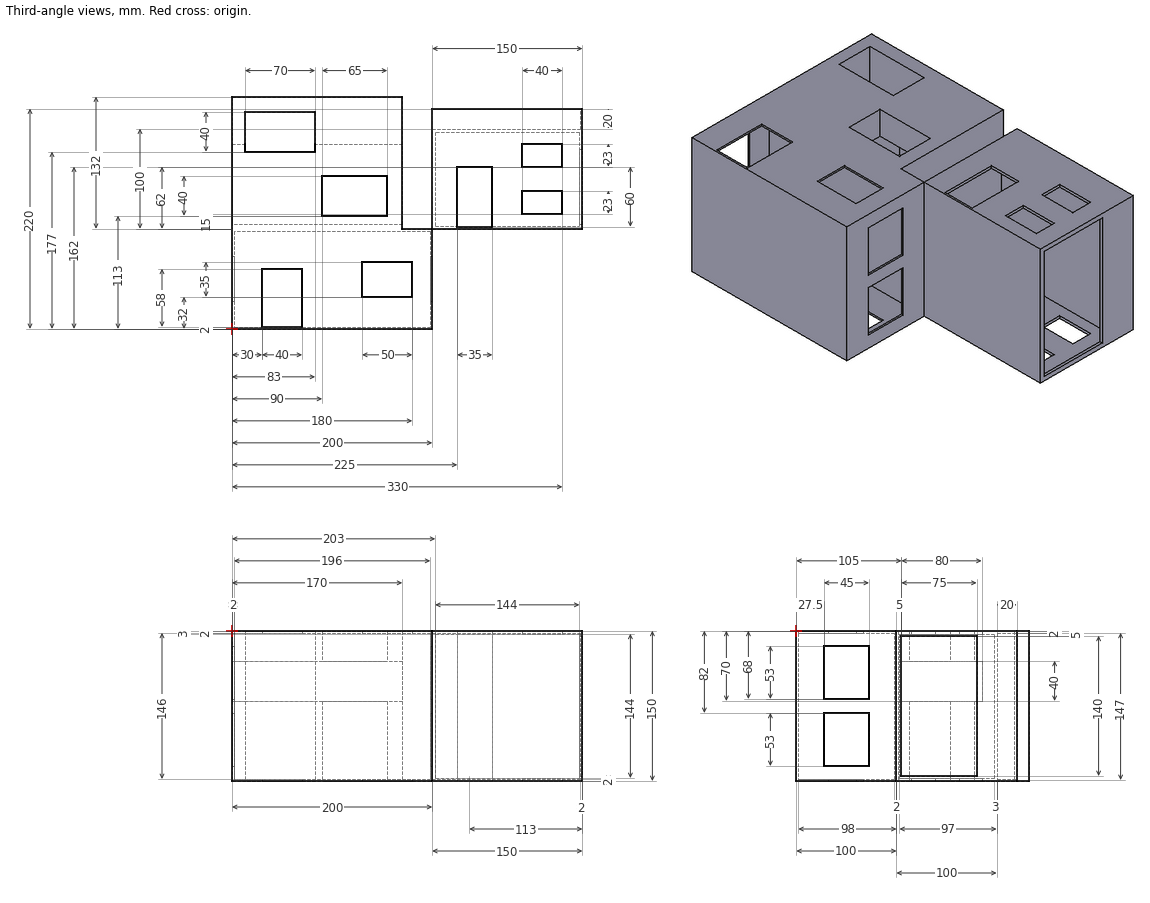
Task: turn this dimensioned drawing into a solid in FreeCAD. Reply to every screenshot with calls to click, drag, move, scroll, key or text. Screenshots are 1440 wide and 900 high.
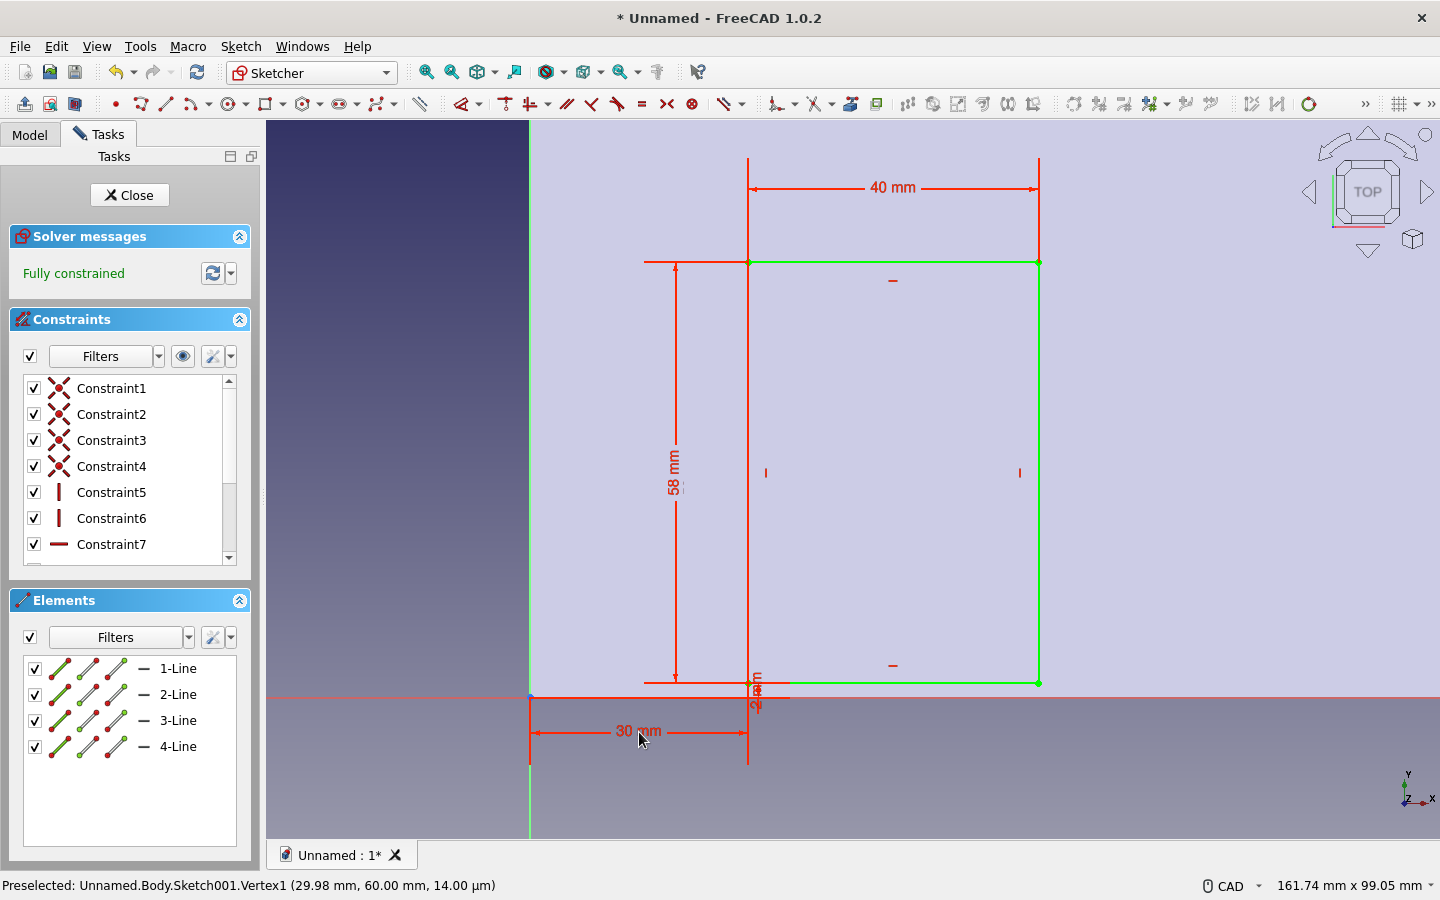
click(130, 195)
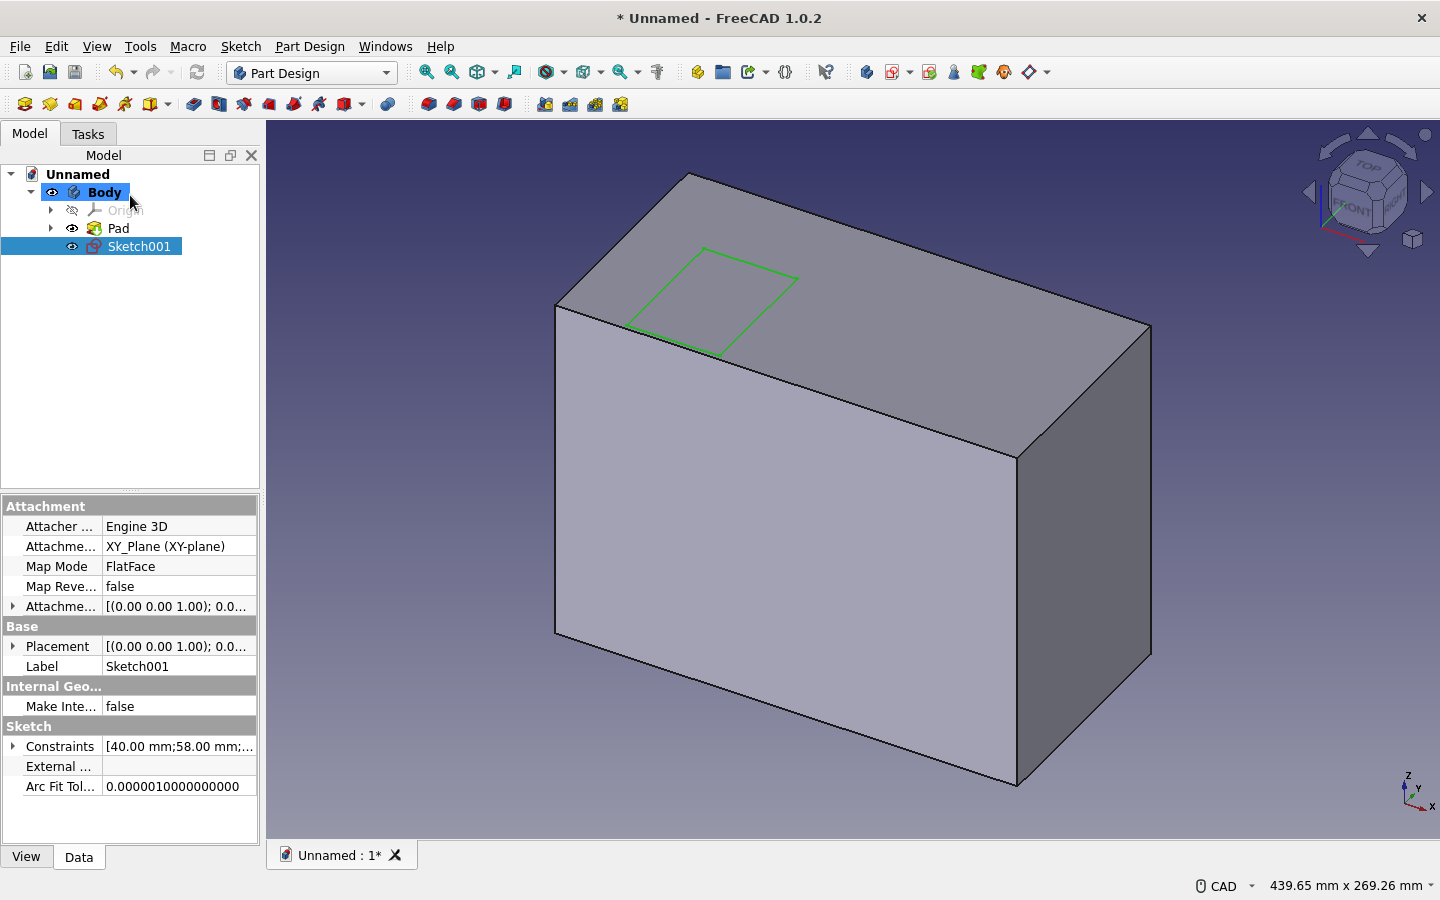
click(194, 104)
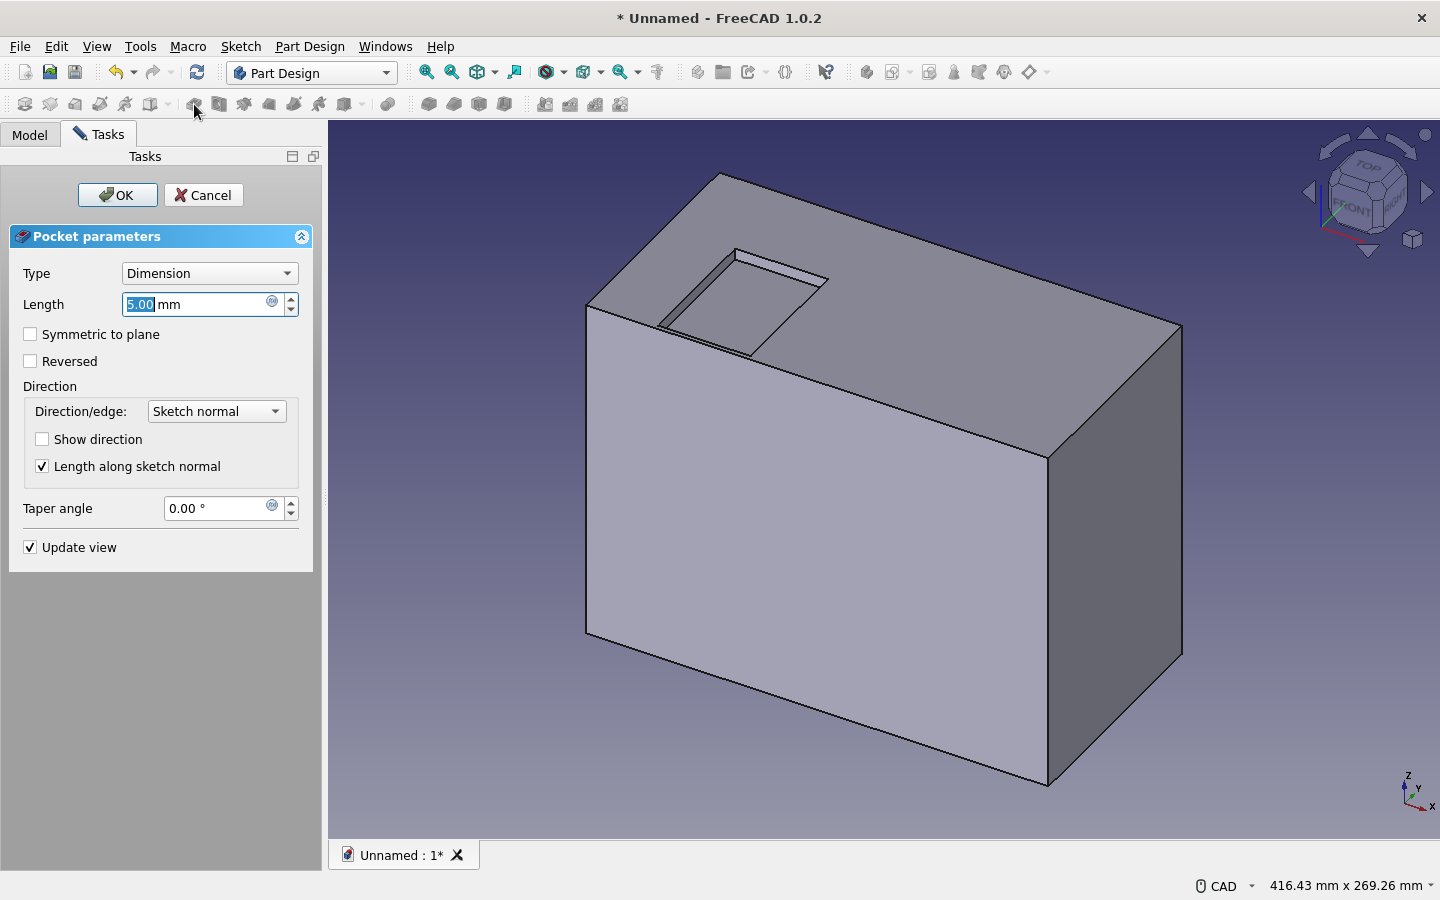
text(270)
key(Tab)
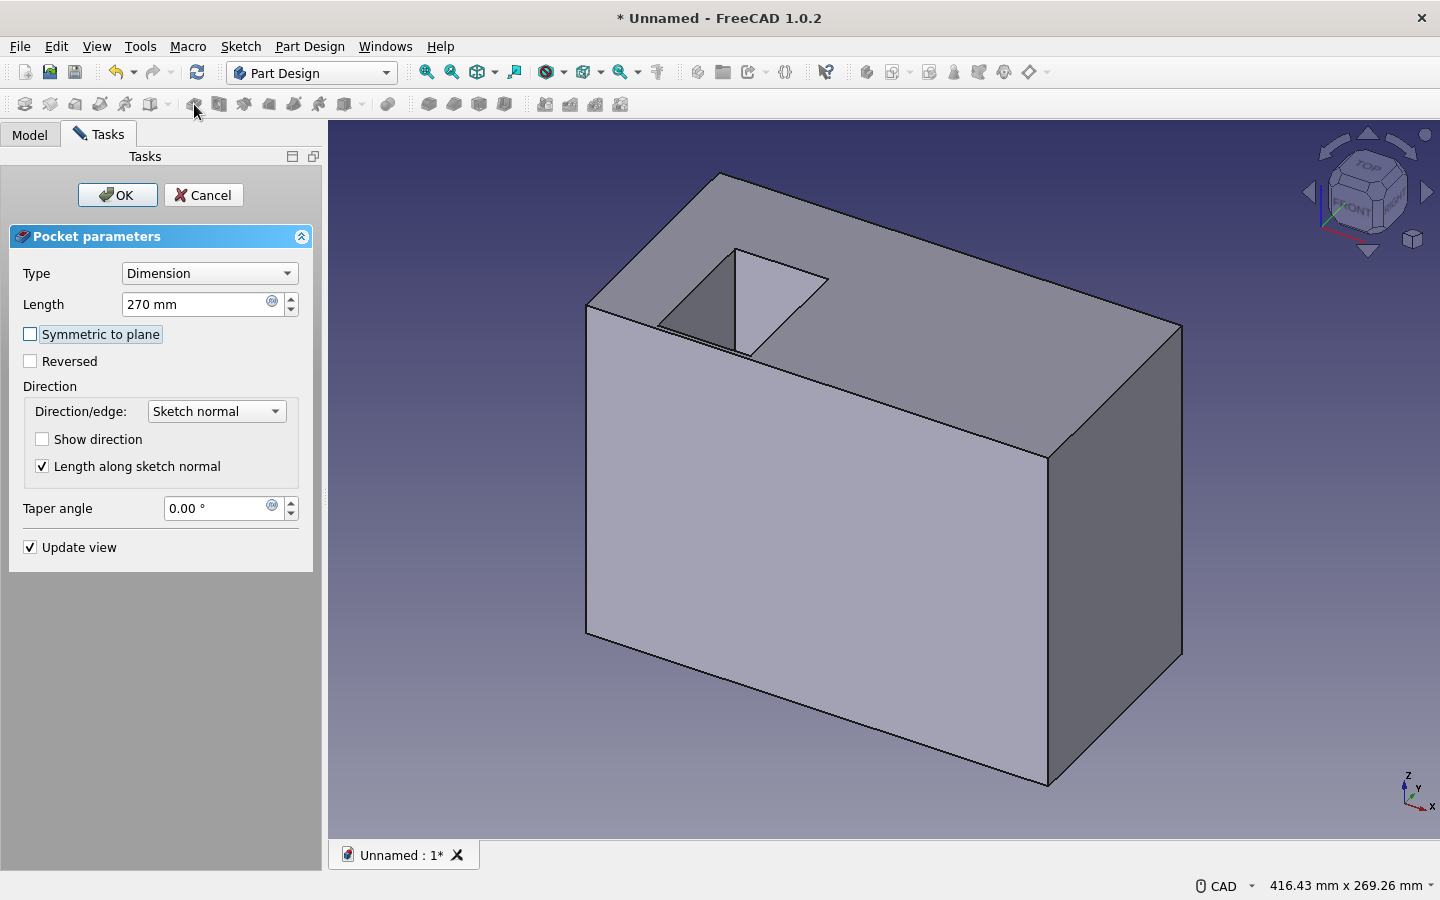
click(118, 195)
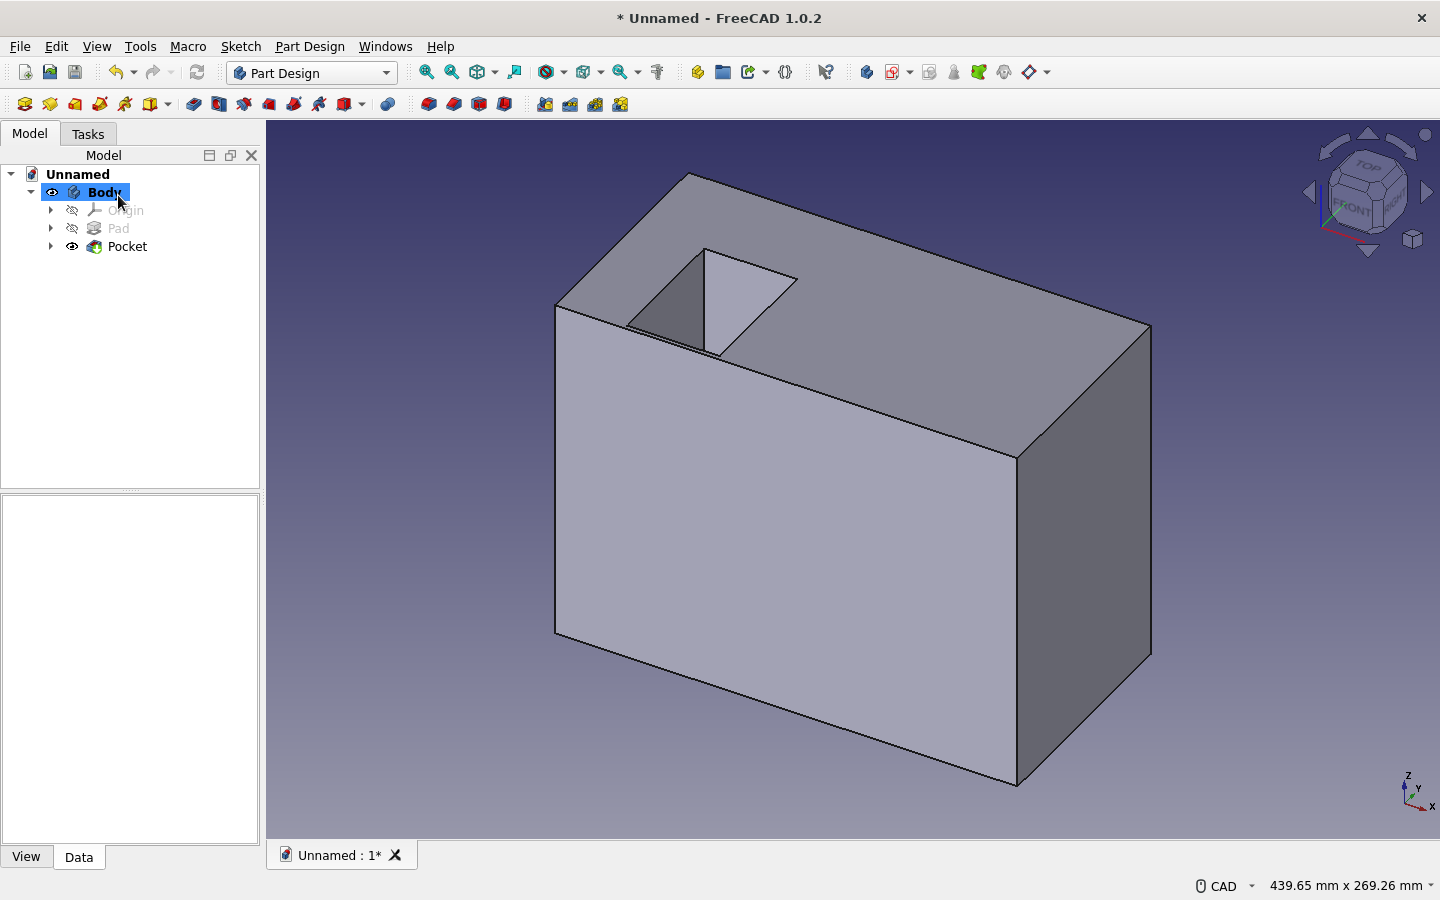
key(4)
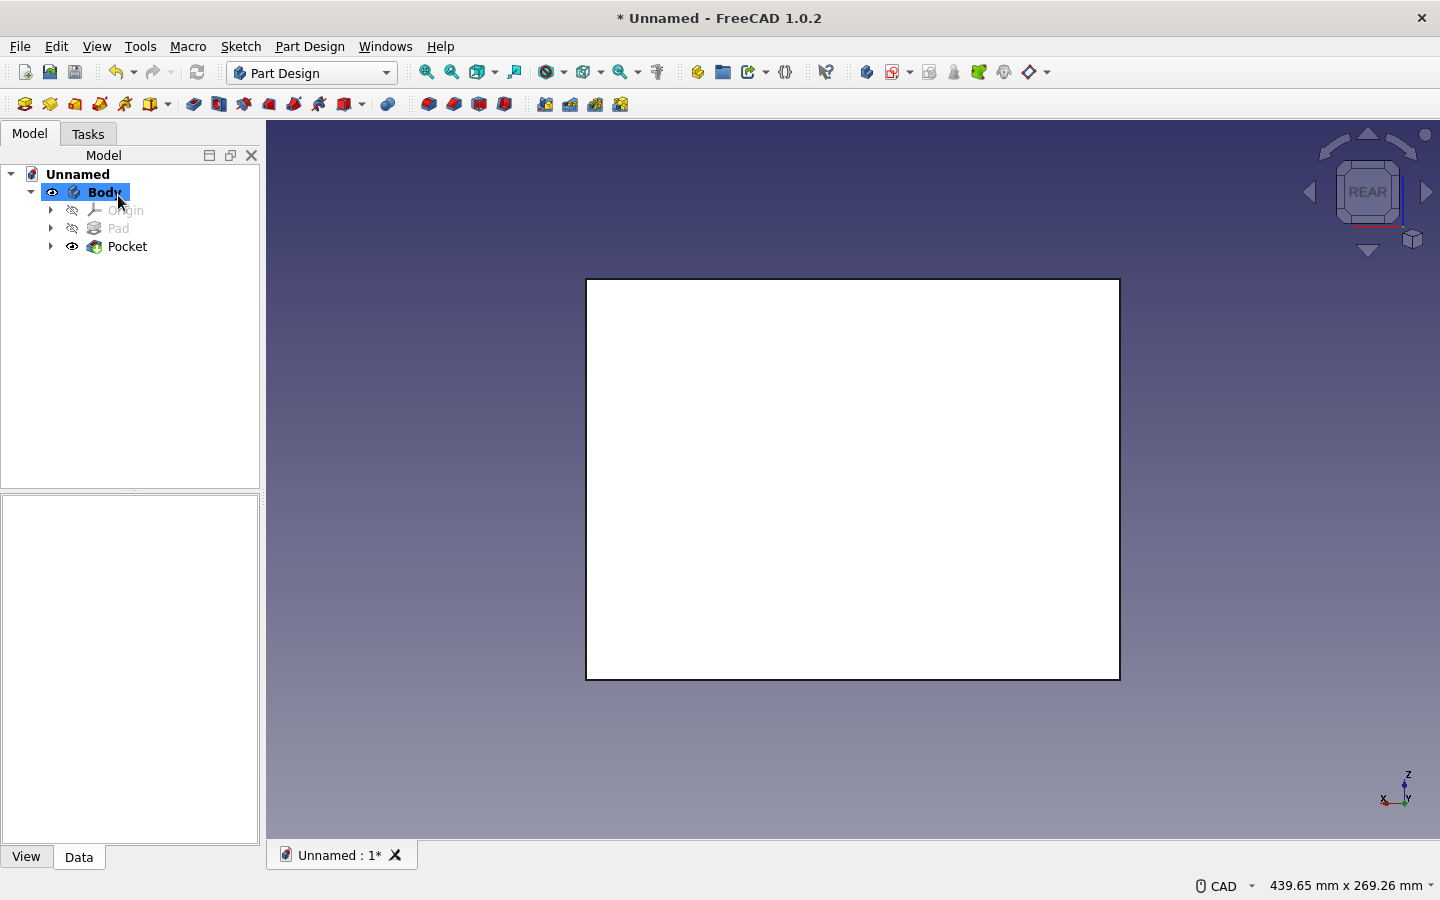
click(853, 479)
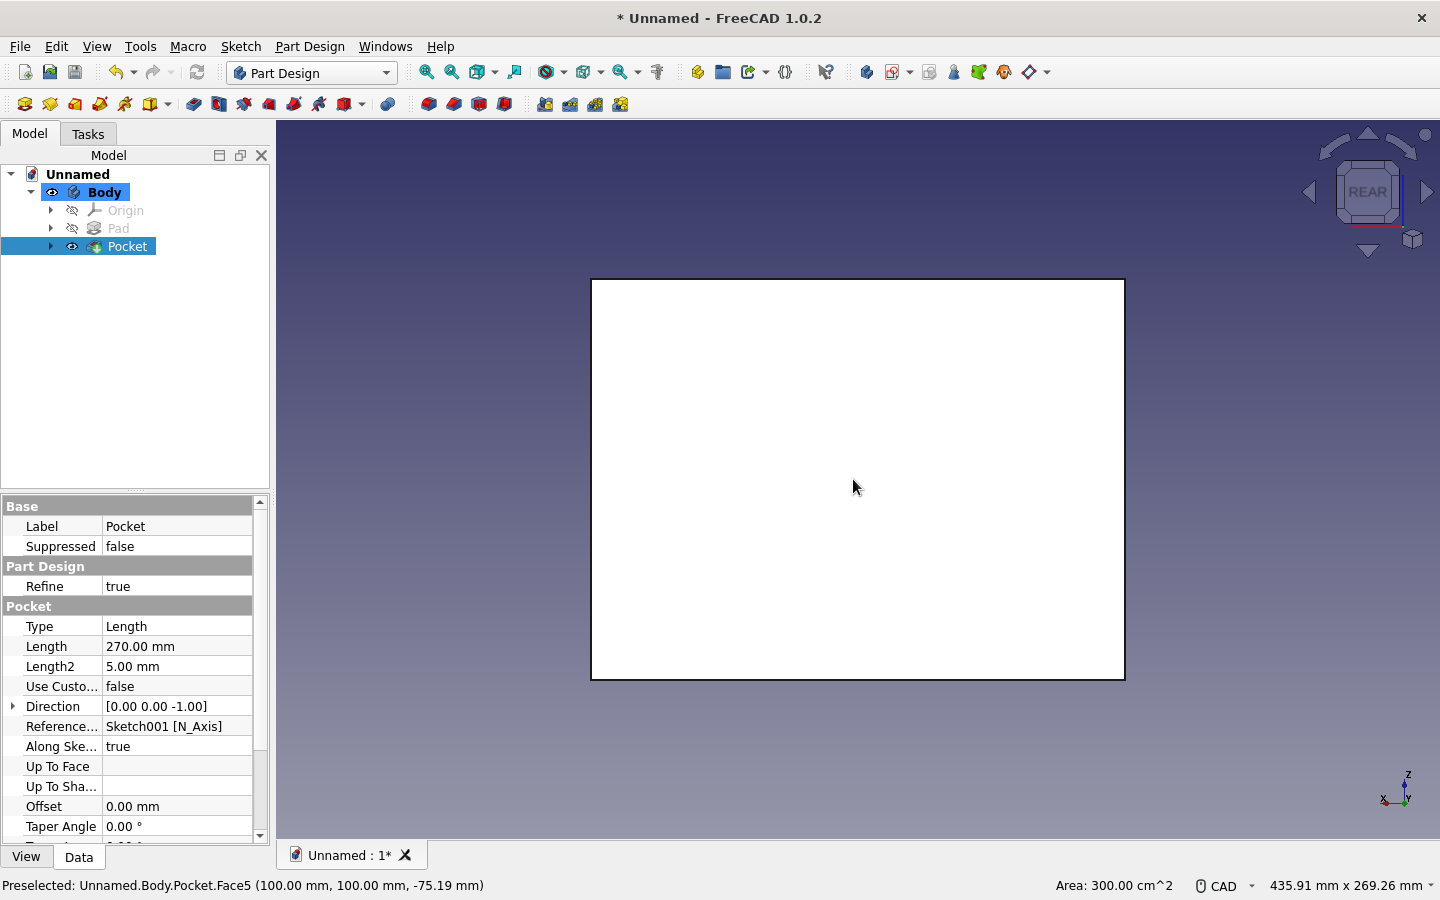
click(892, 72)